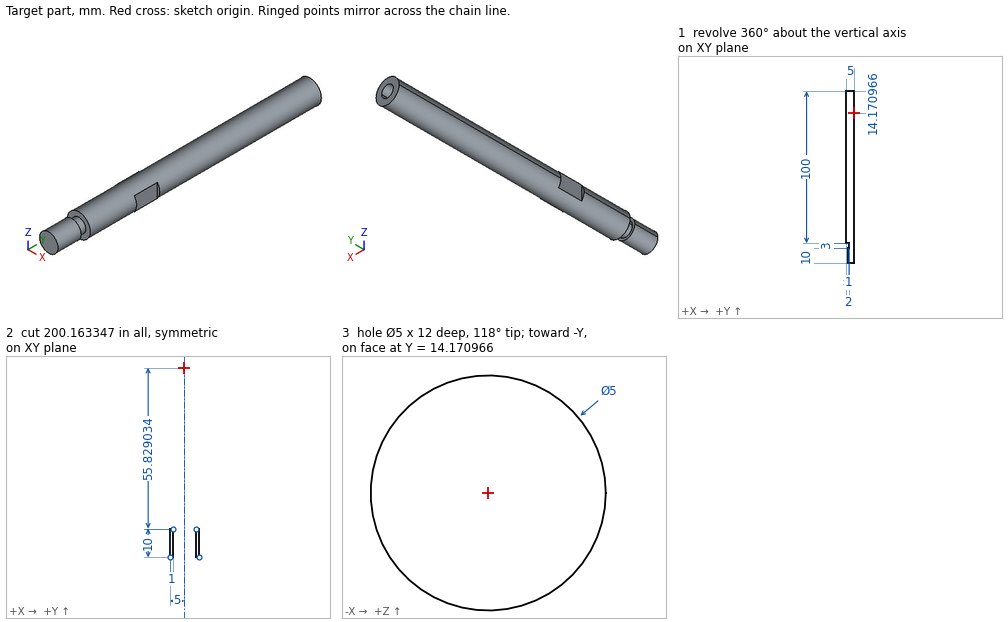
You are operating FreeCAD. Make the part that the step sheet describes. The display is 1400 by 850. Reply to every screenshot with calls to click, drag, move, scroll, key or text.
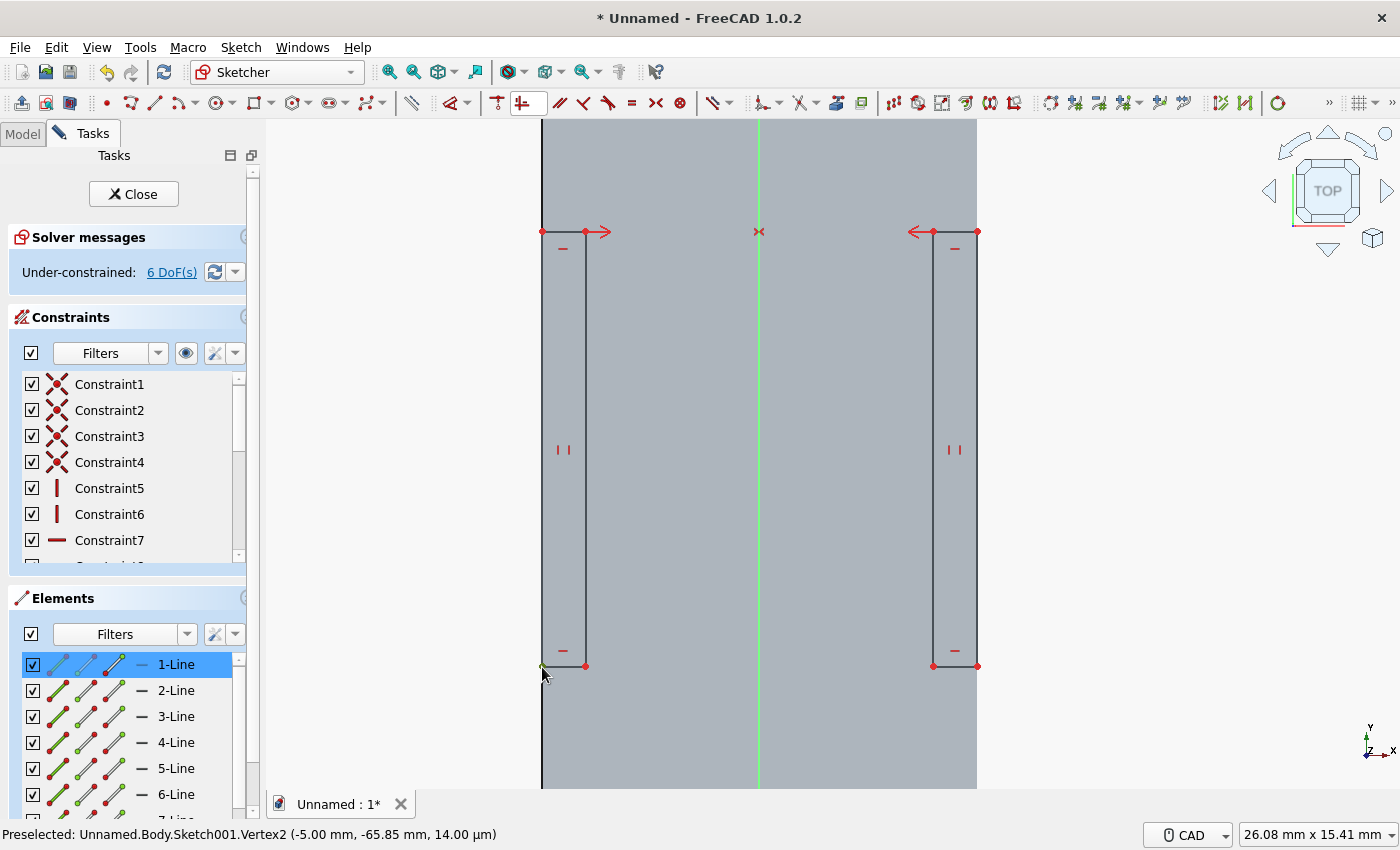
click(977, 667)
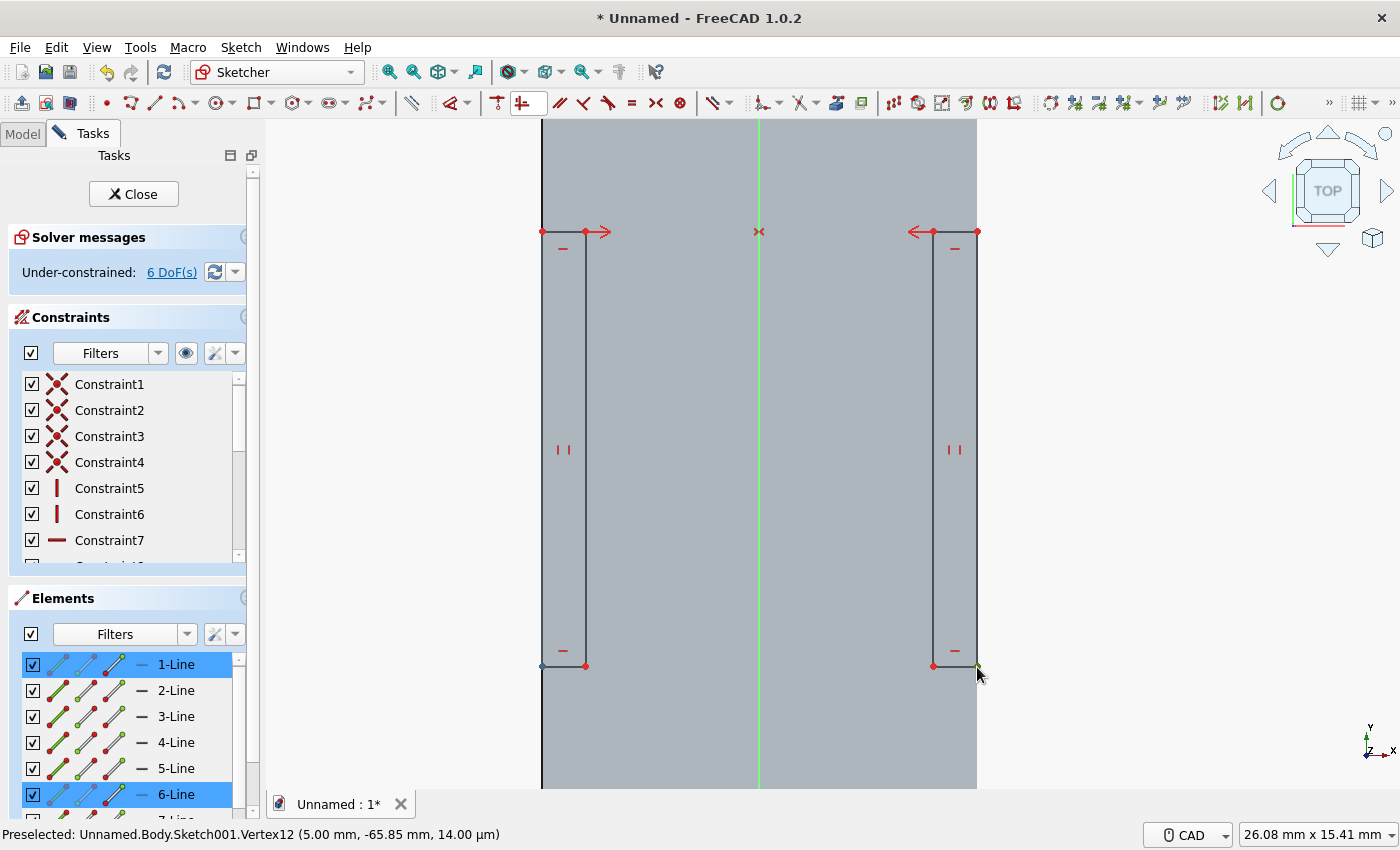
click(759, 717)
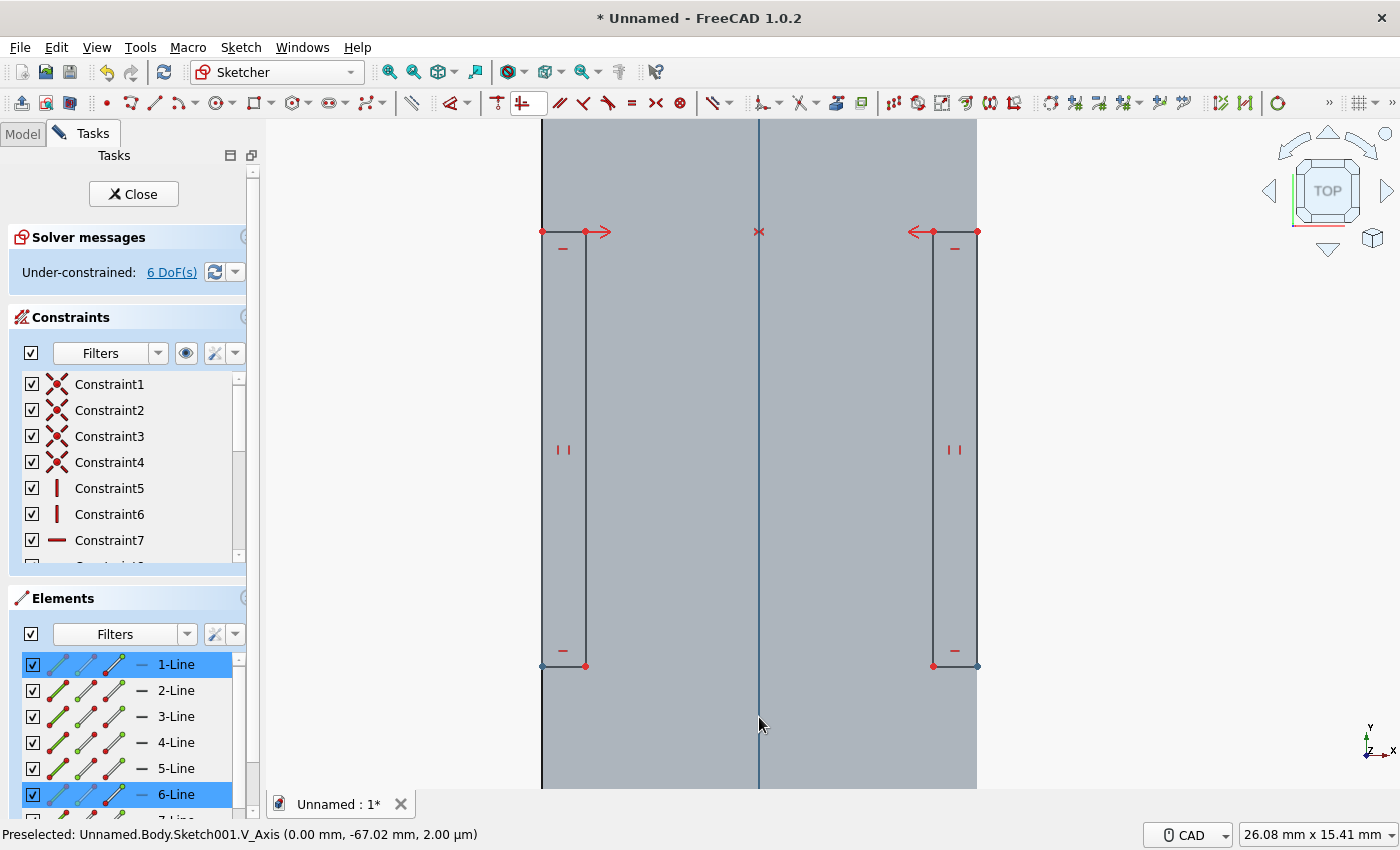
click(656, 104)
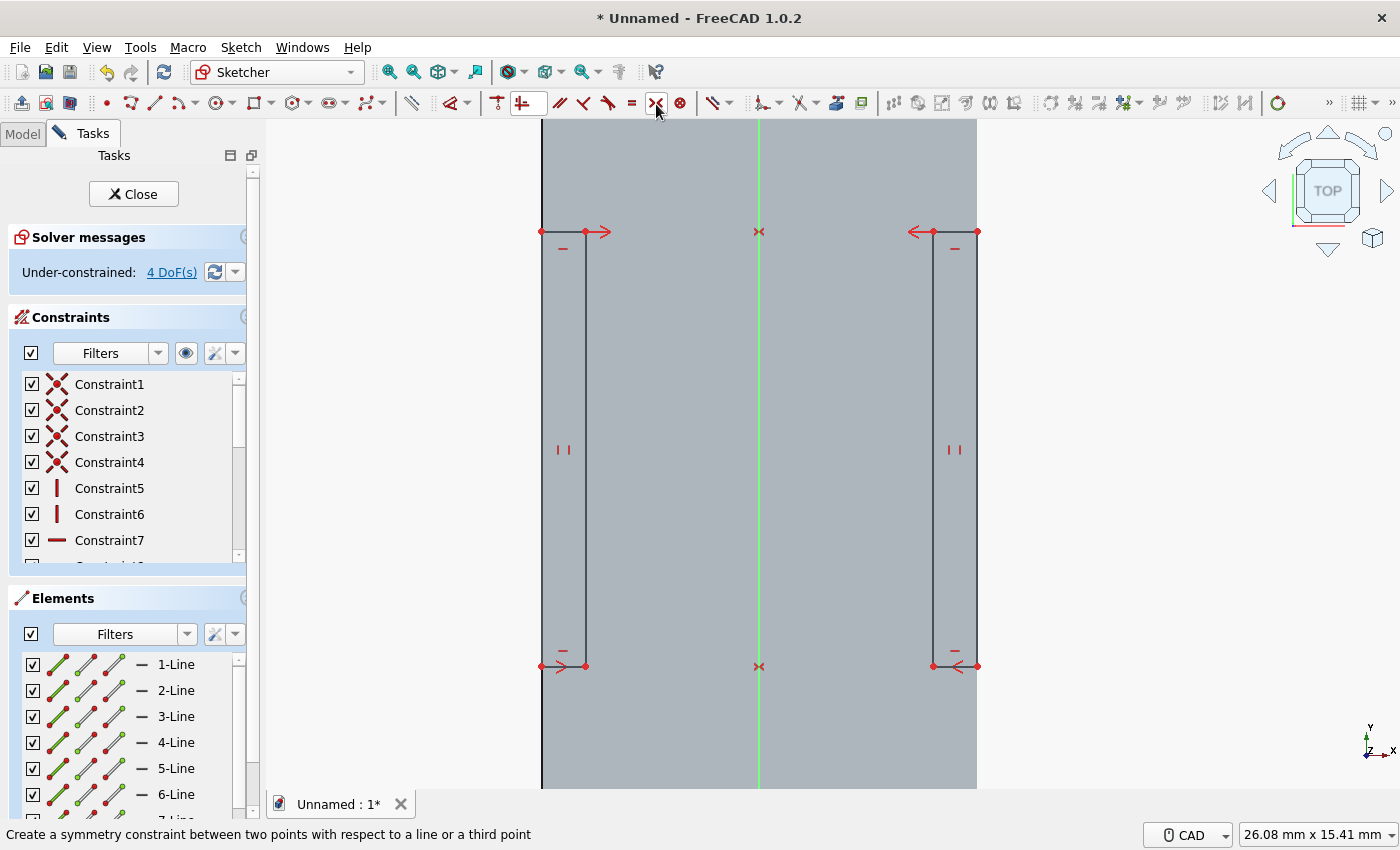
click(450, 104)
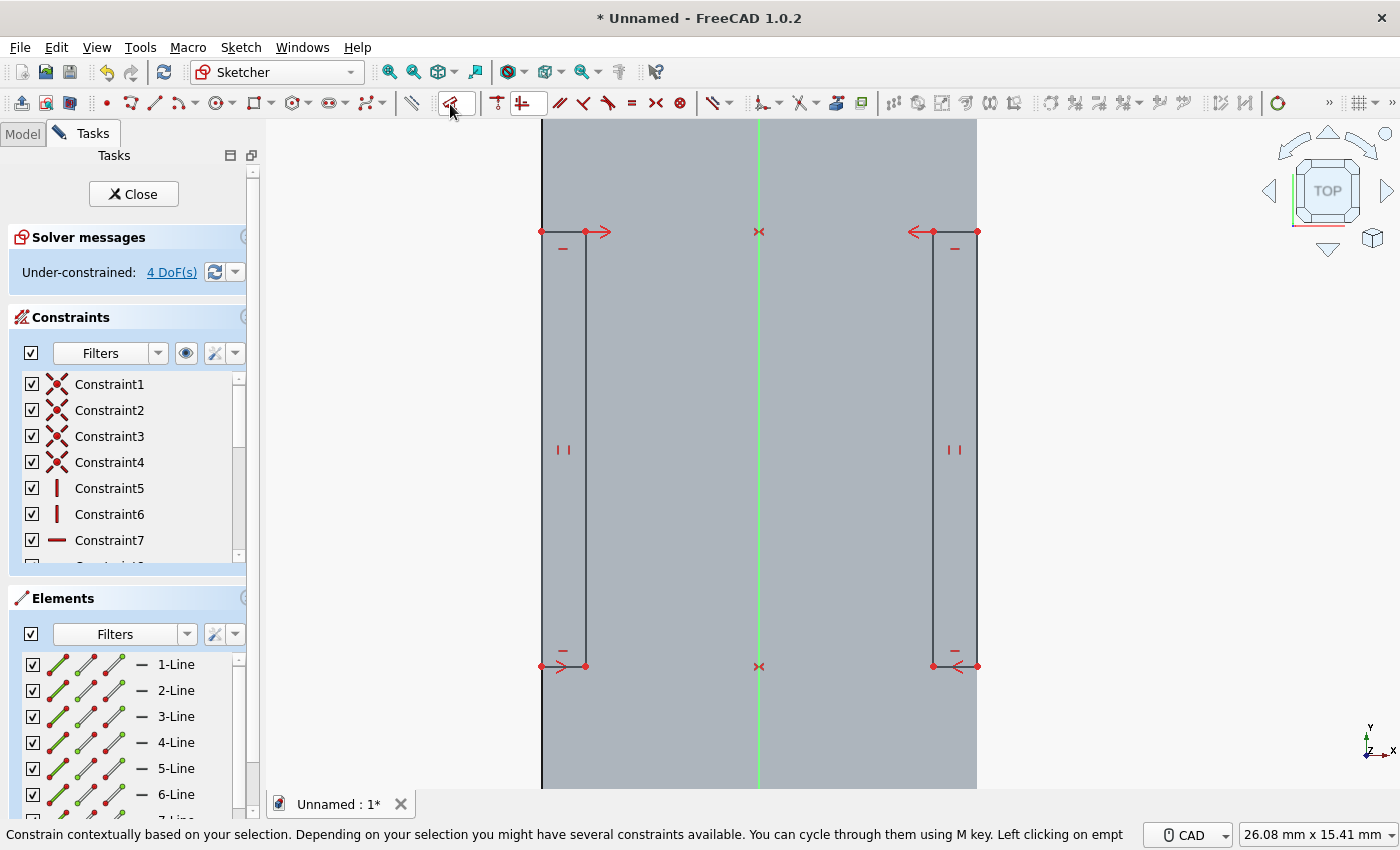
click(555, 667)
click(564, 701)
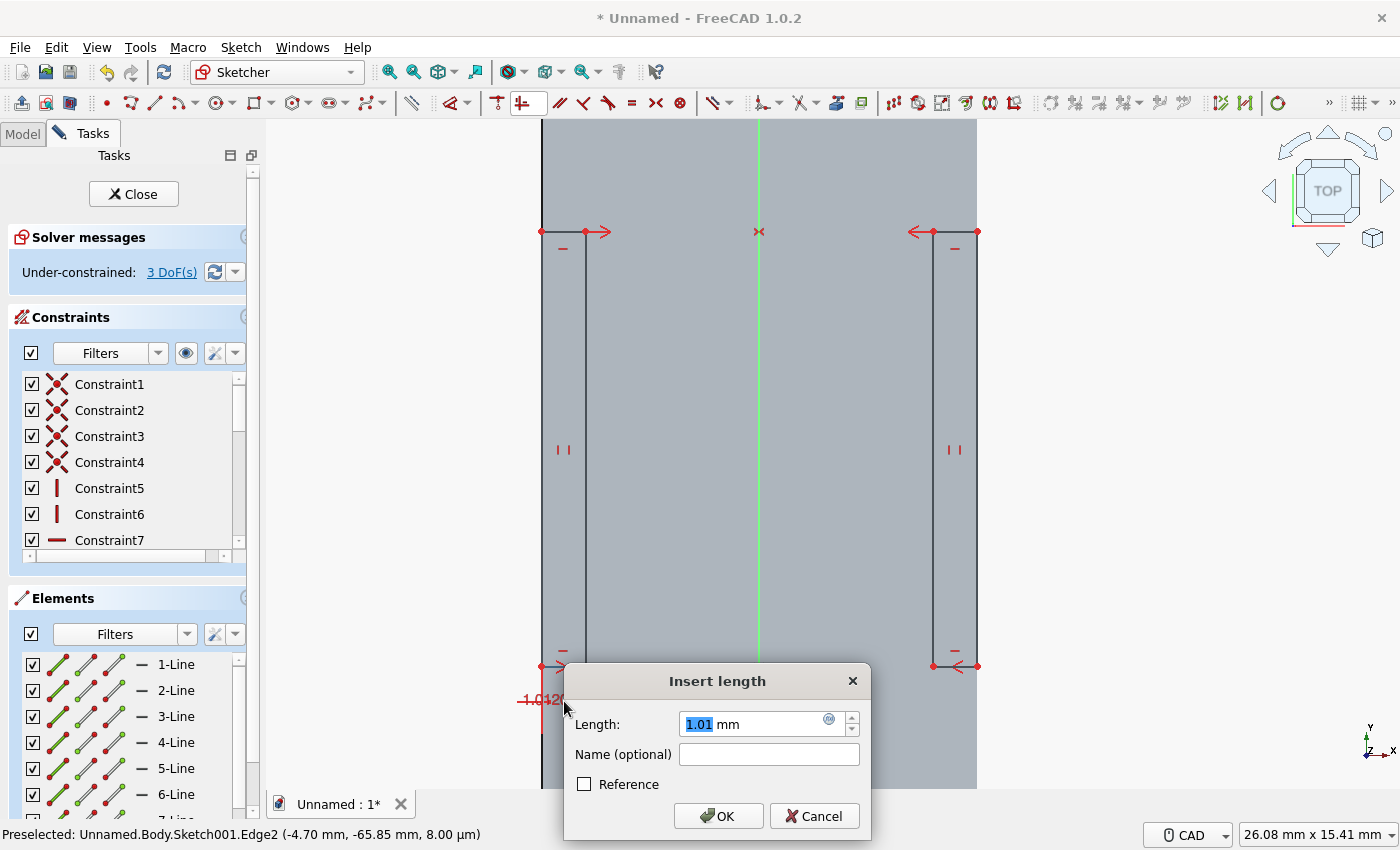
text(1)
key(Return)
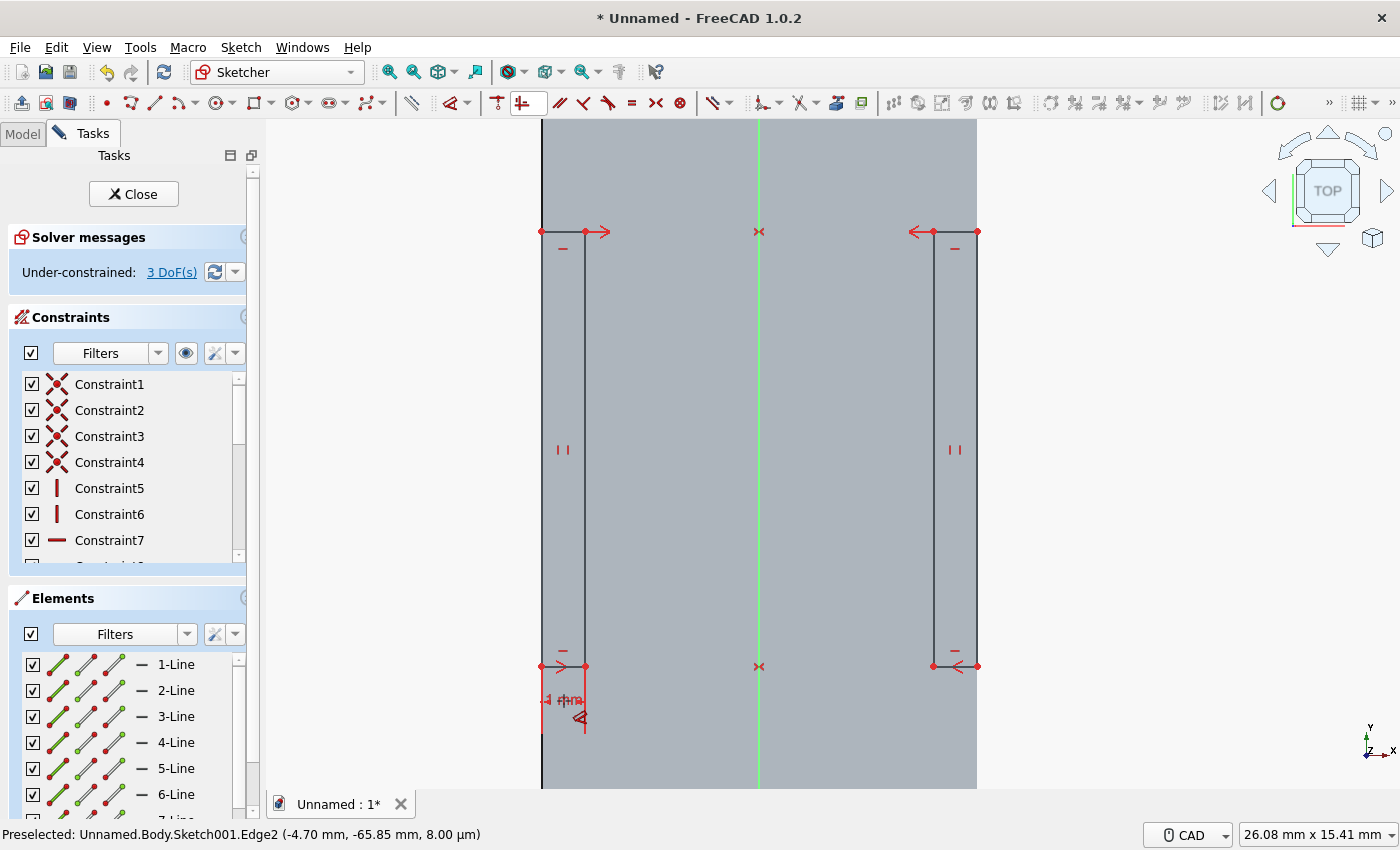
click(542, 362)
click(508, 449)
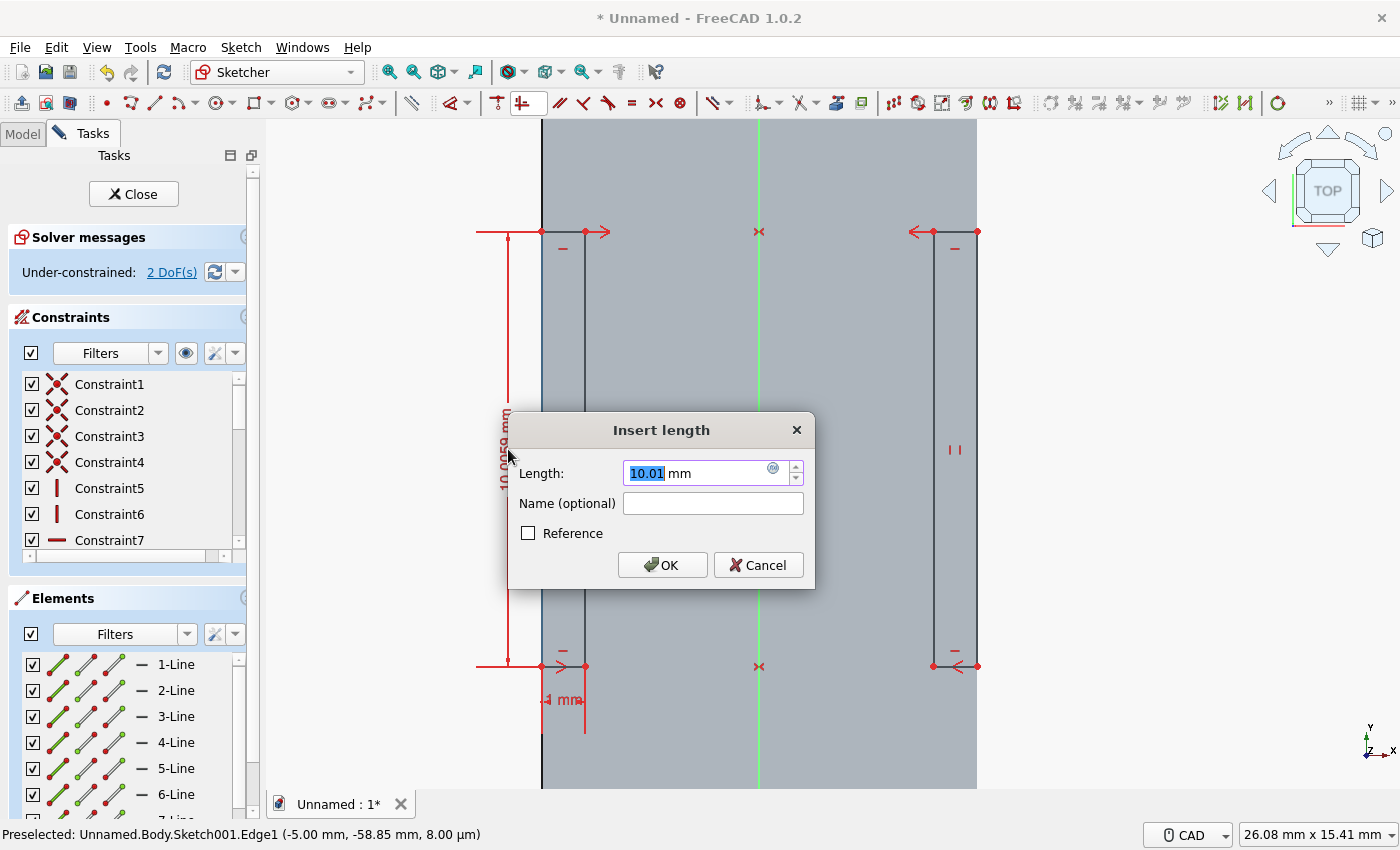
text(10)
key(Return)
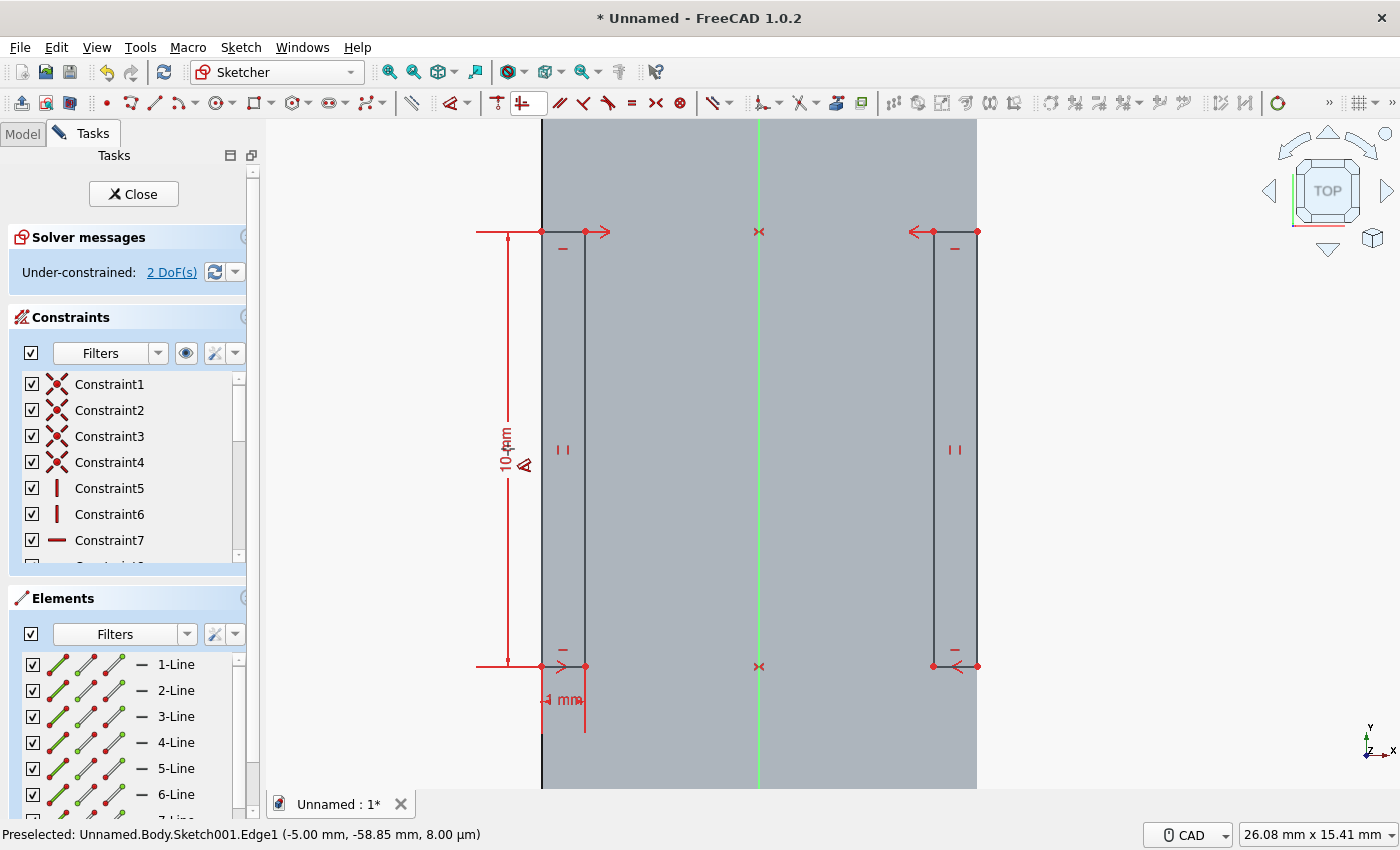
click(542, 232)
click(651, 266)